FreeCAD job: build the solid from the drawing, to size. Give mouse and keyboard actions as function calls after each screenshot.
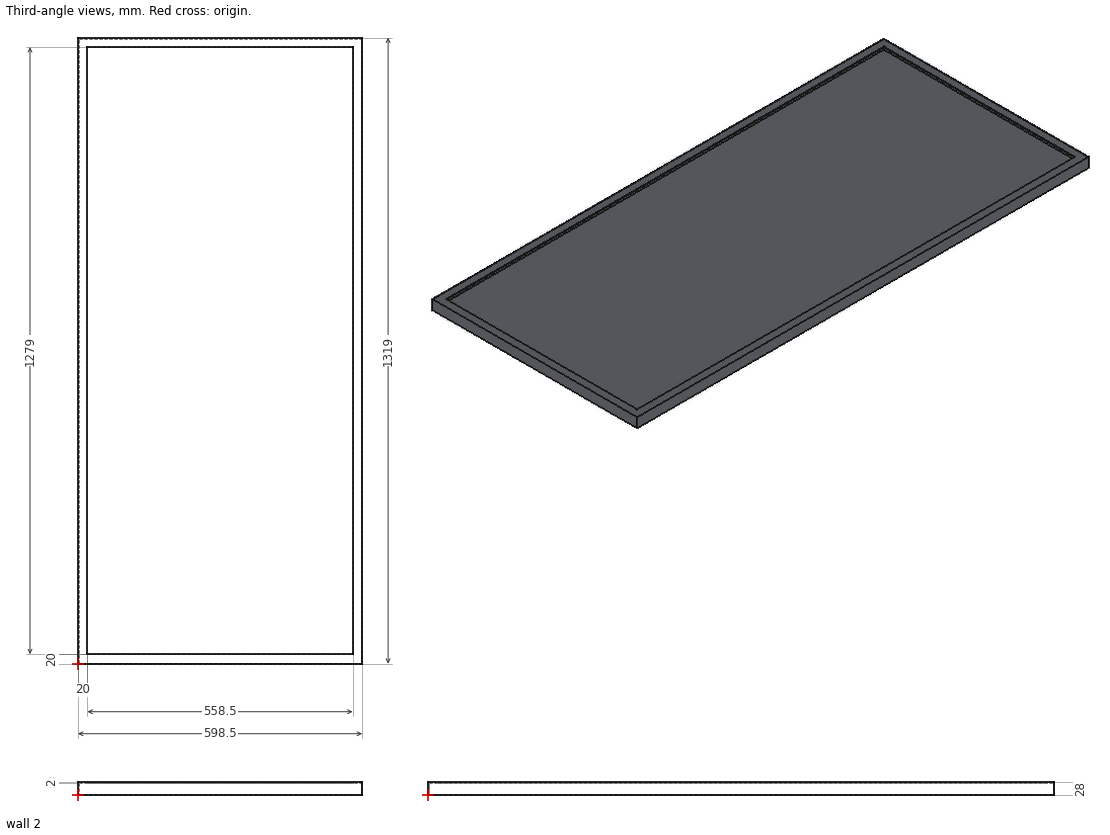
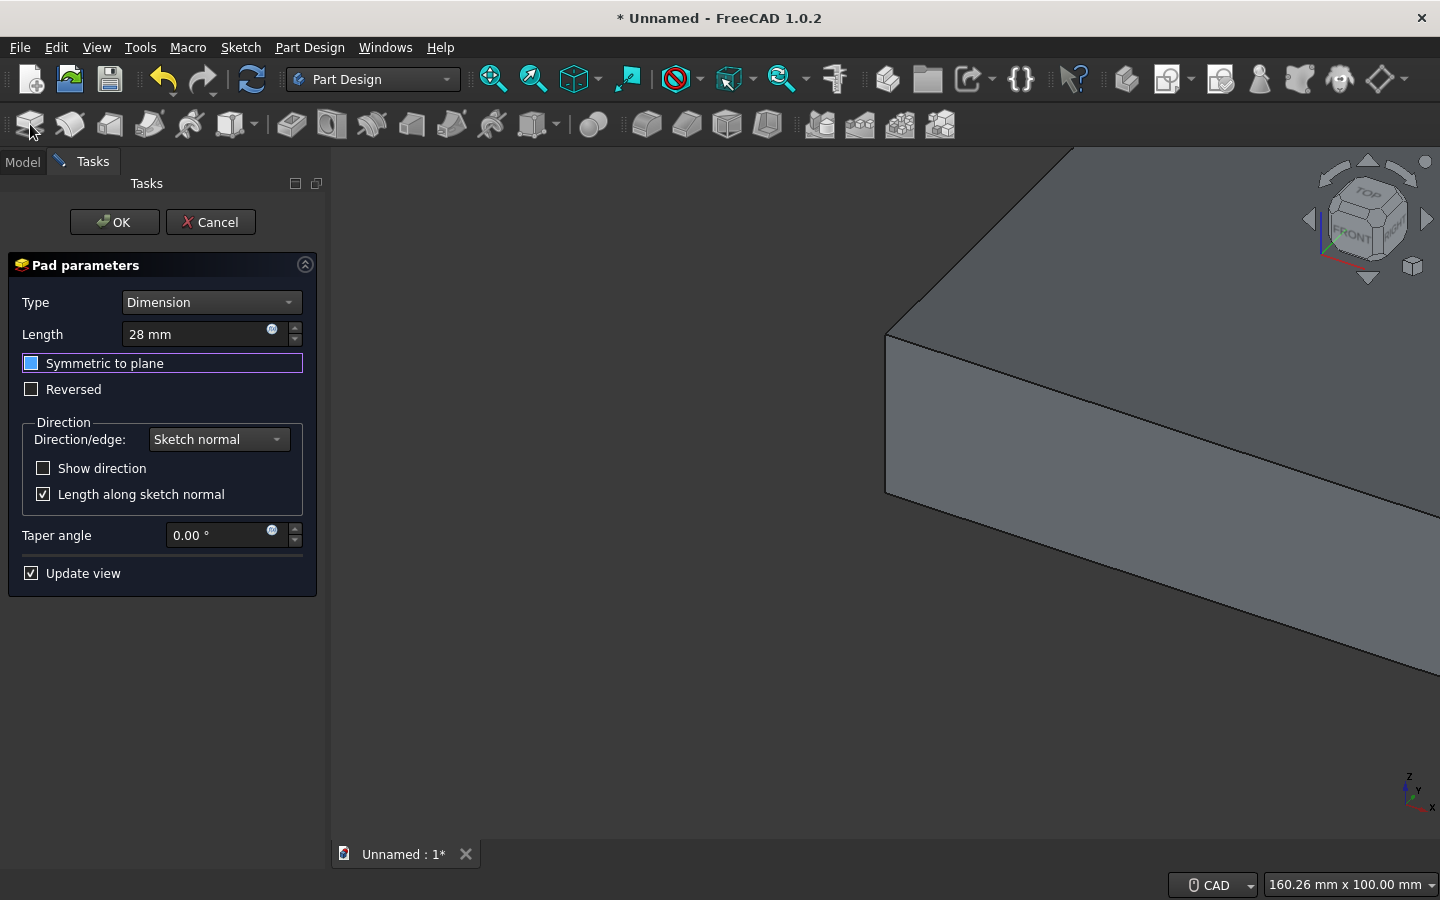
click(115, 222)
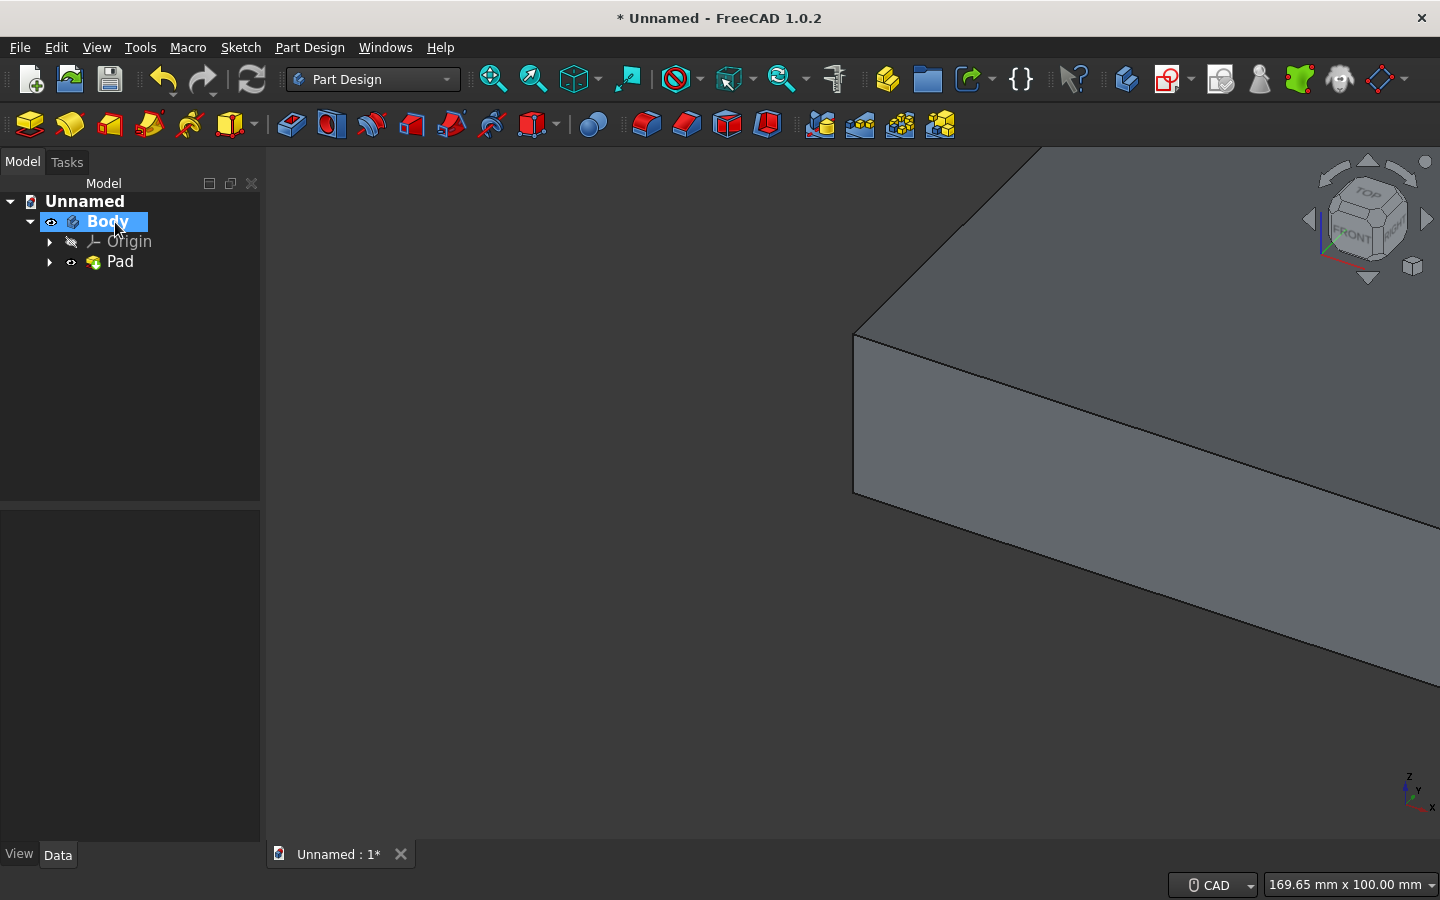
key(v)
key(f)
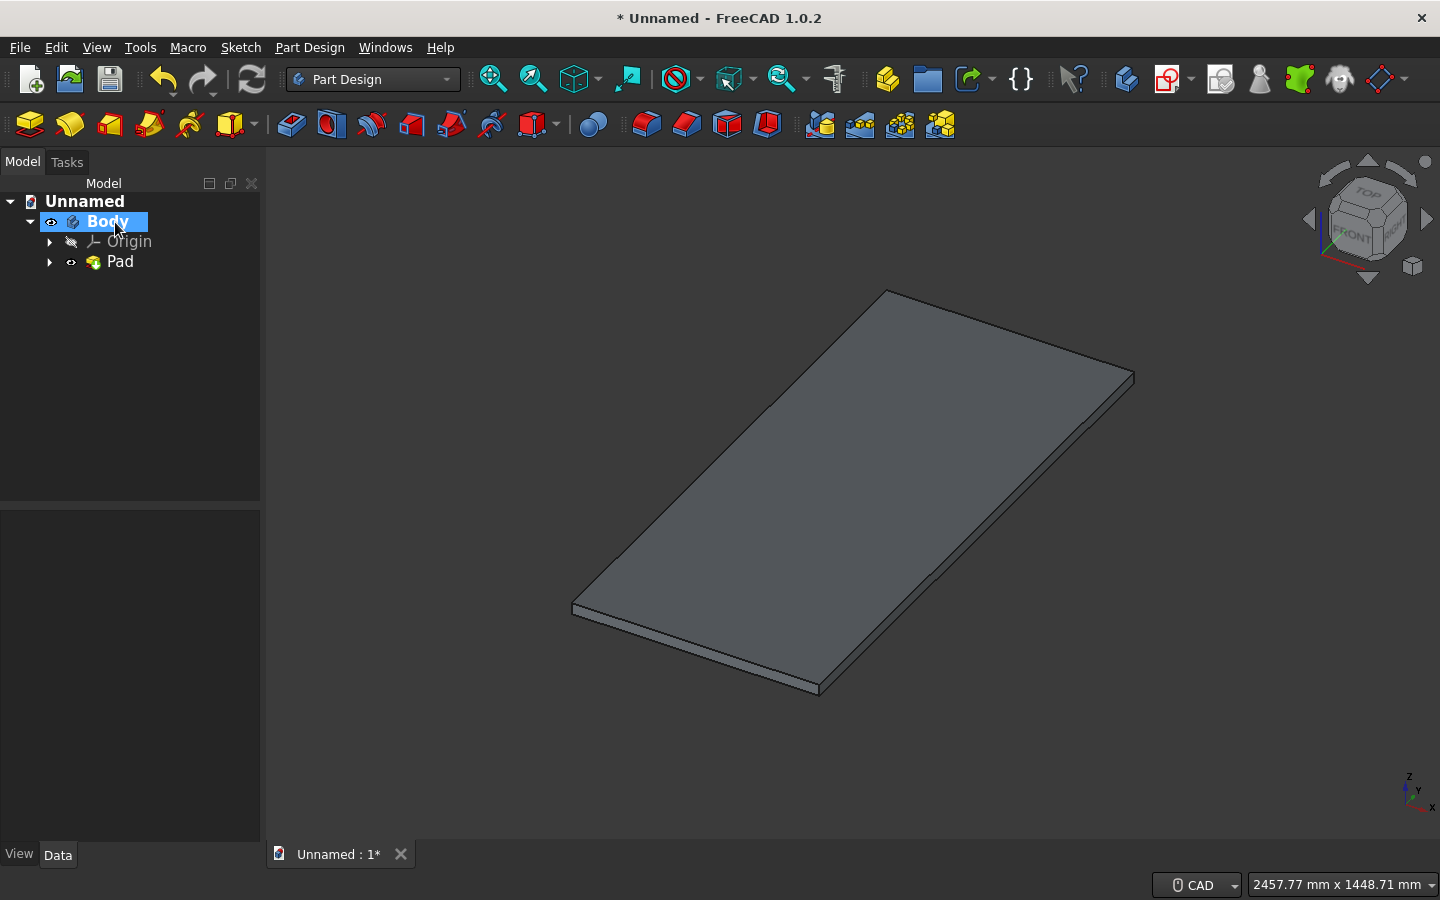
click(898, 442)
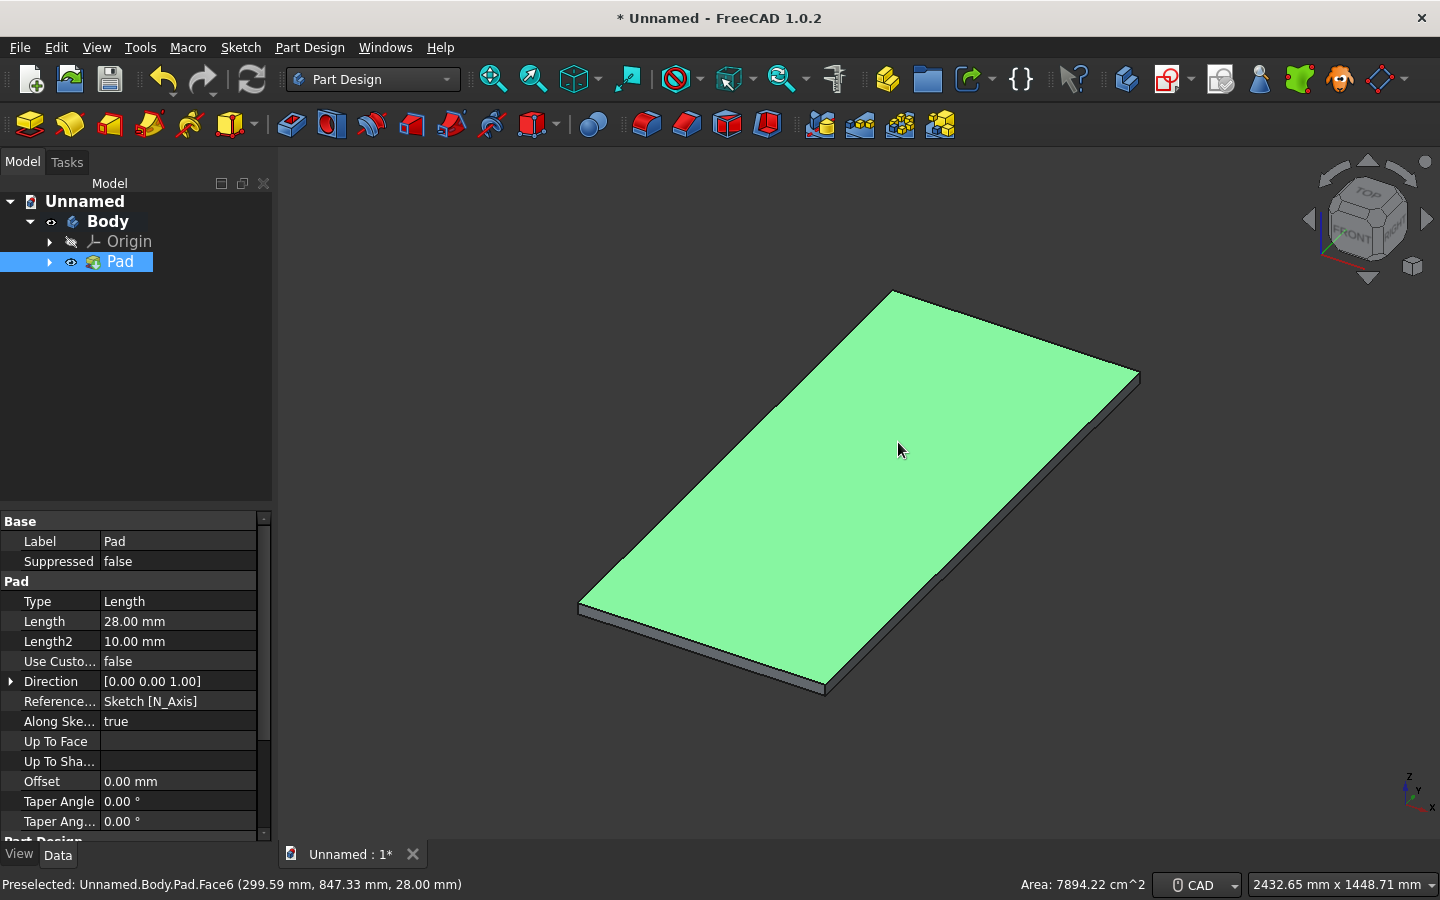
click(768, 124)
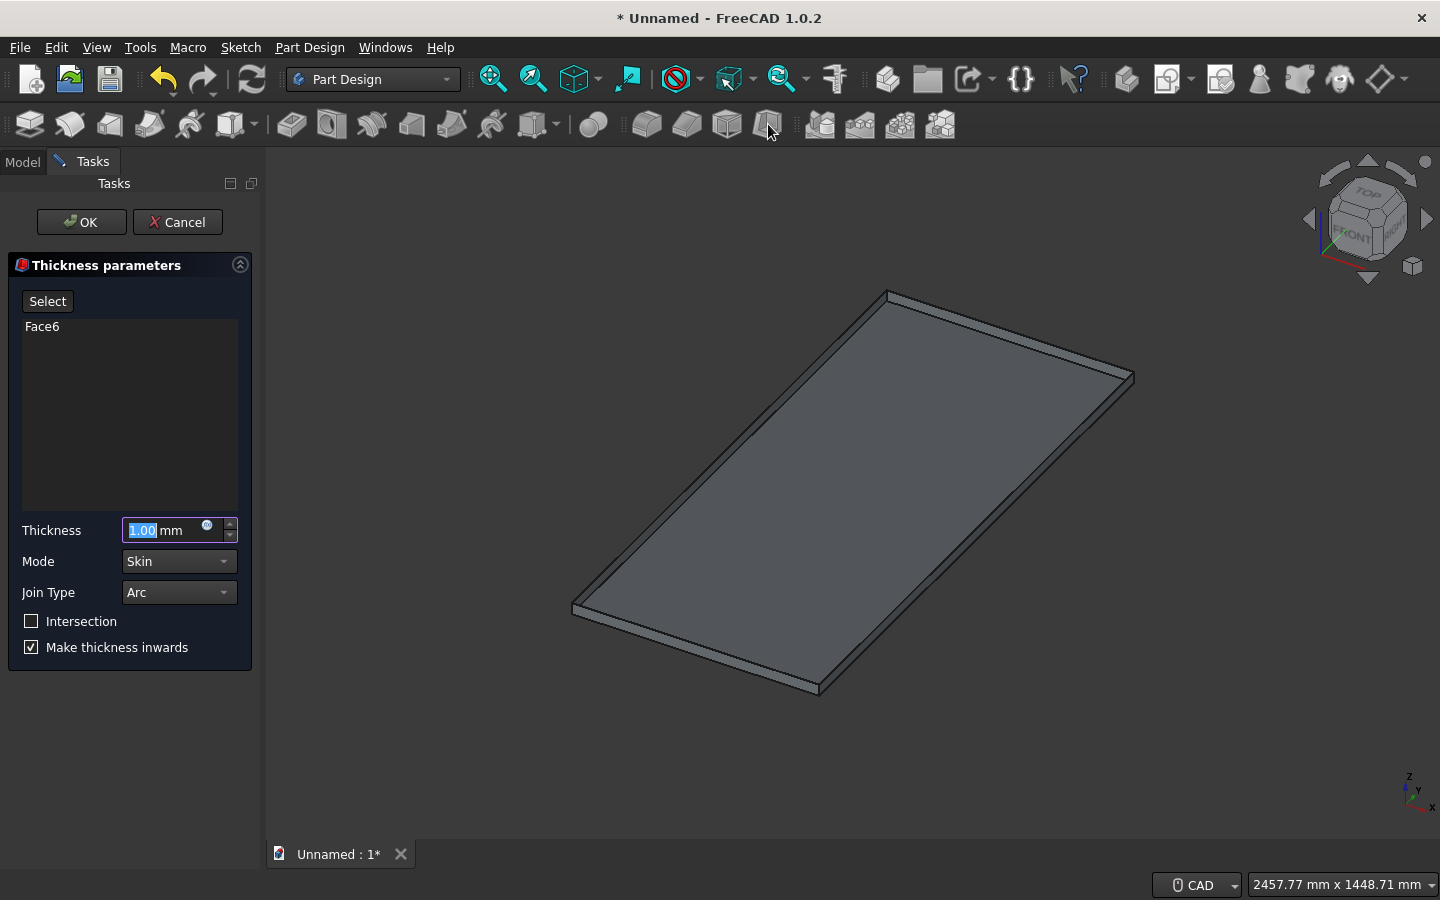
text(2)
key(Tab)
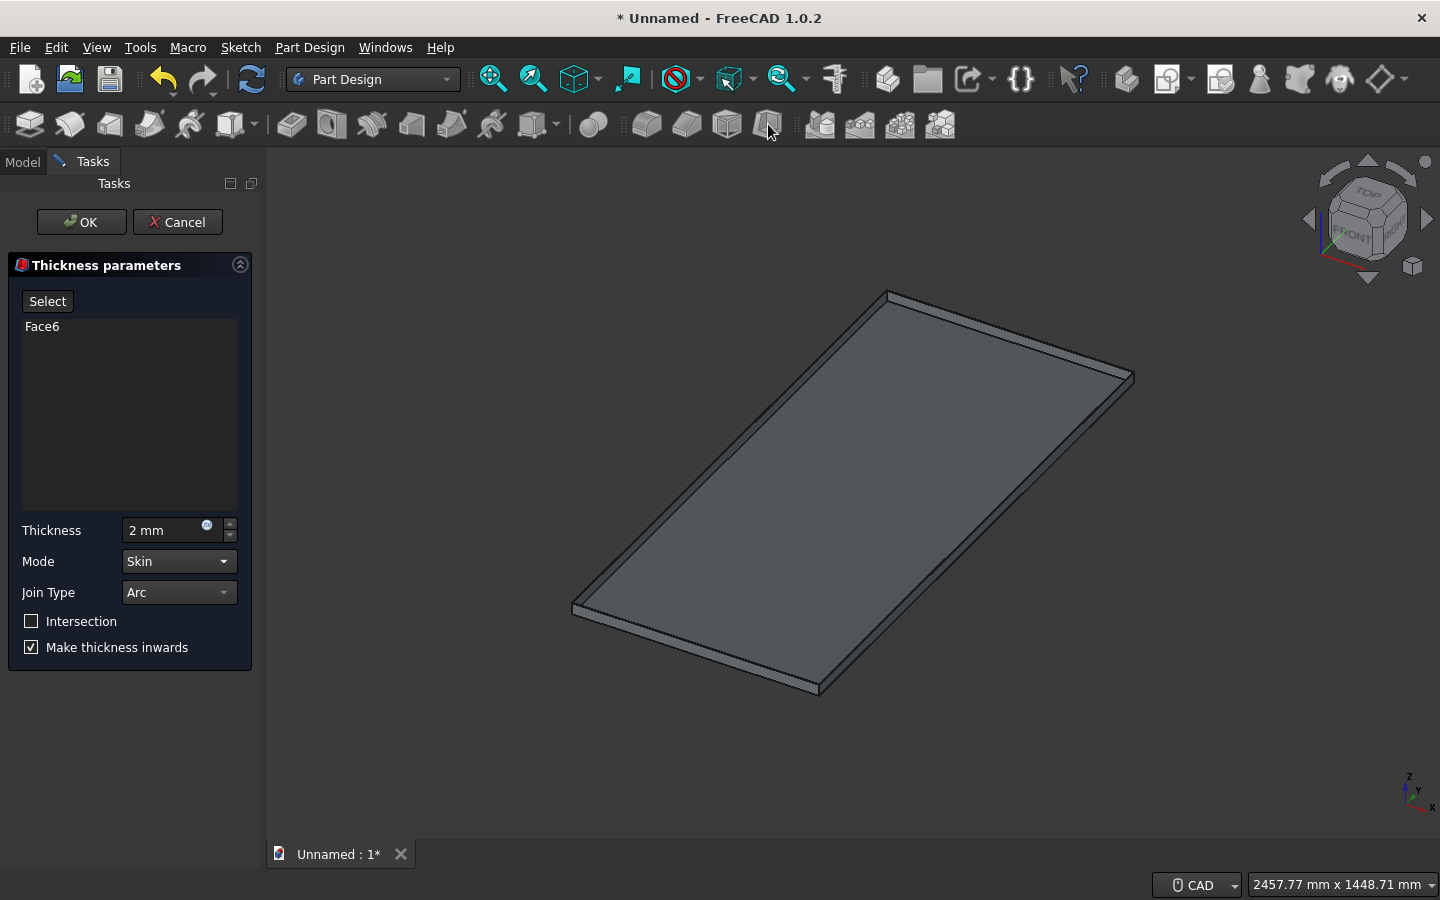
click(180, 592)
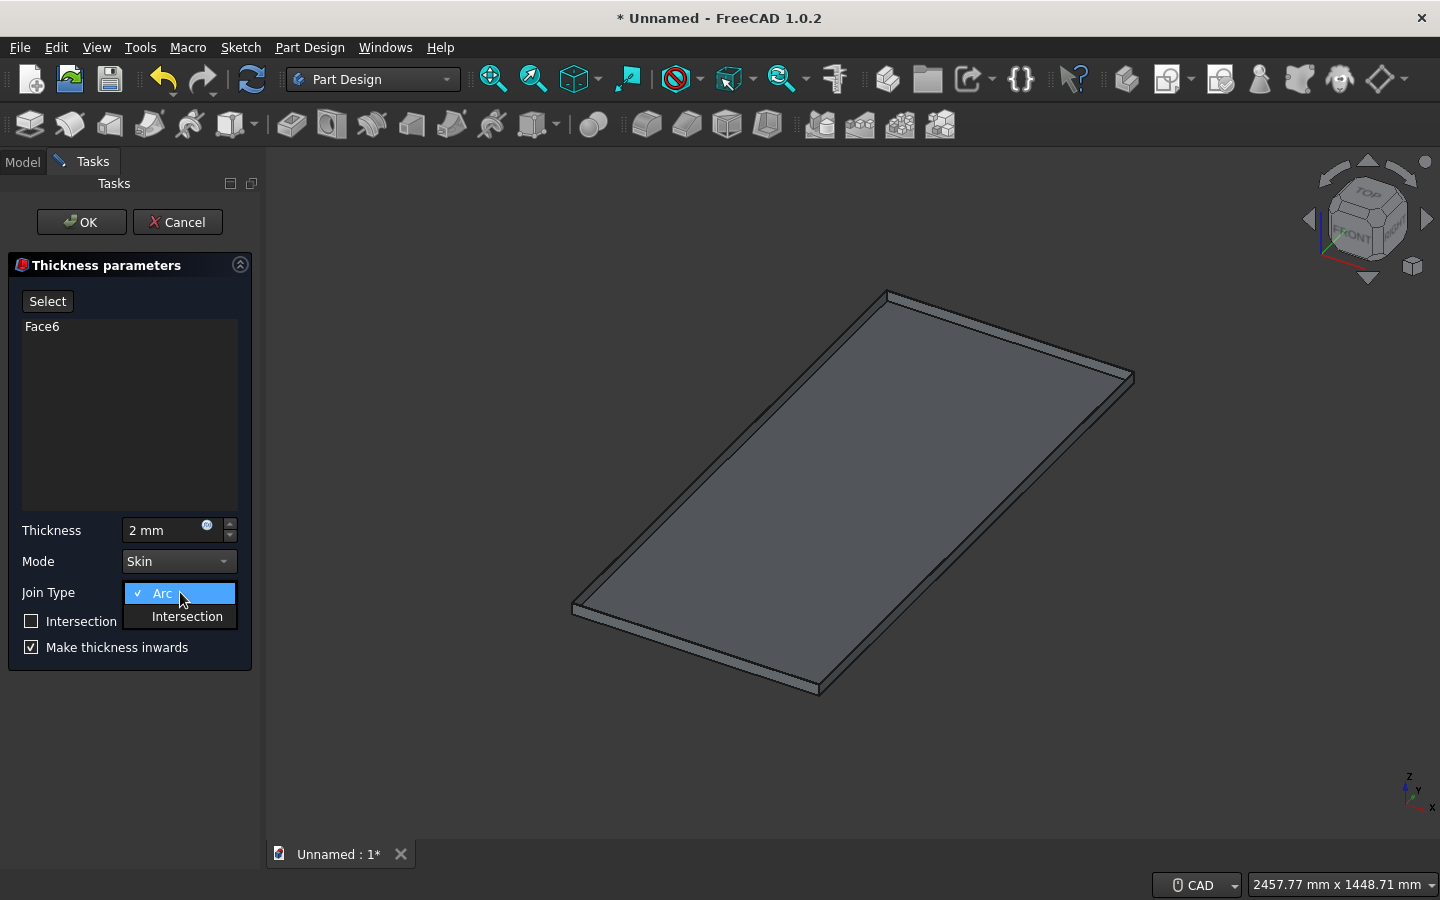
click(179, 616)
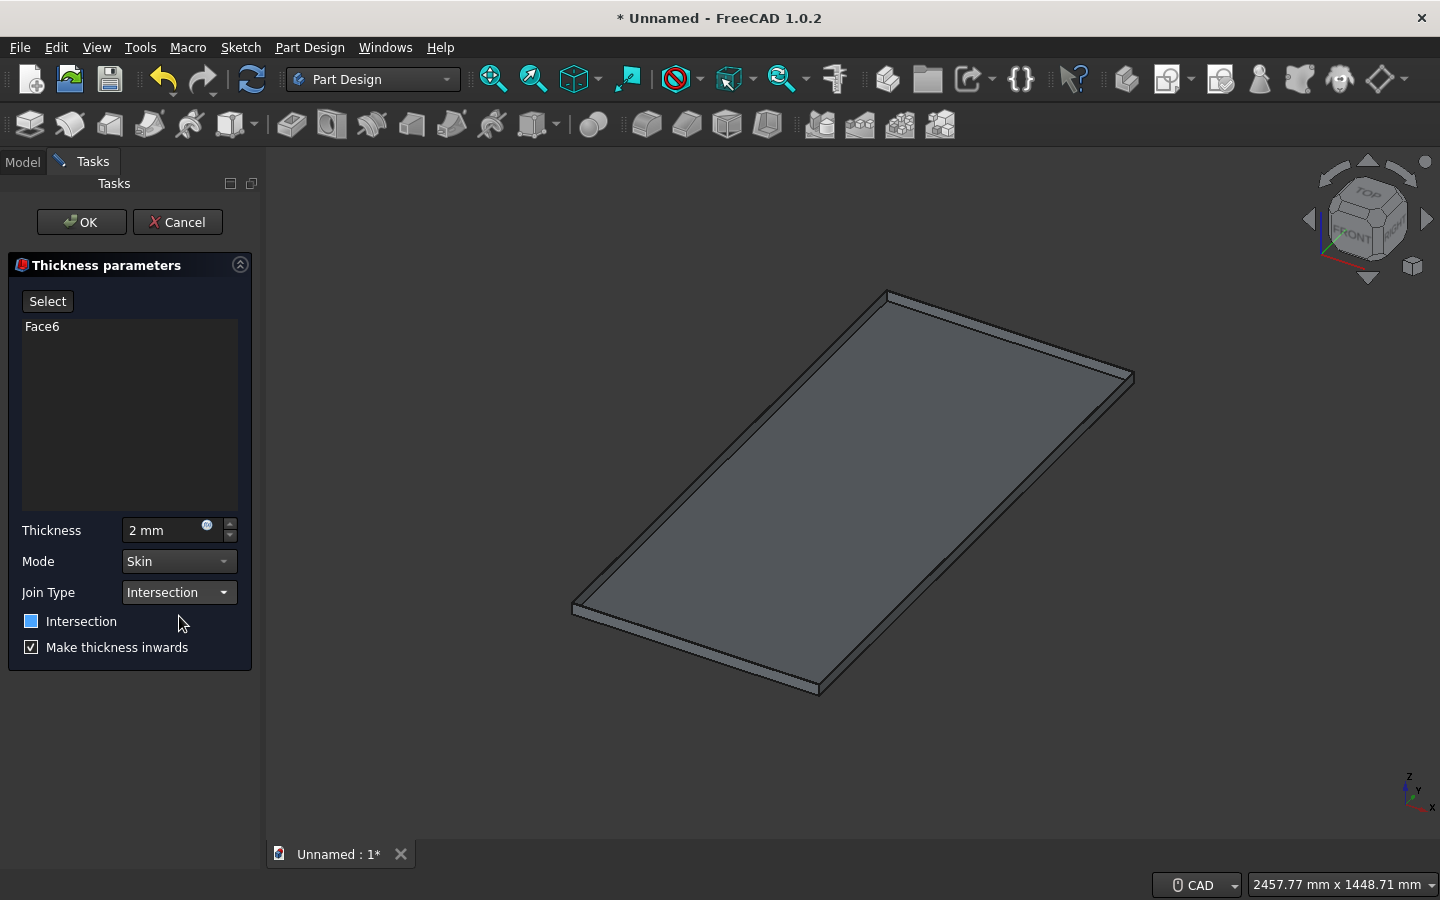
click(82, 222)